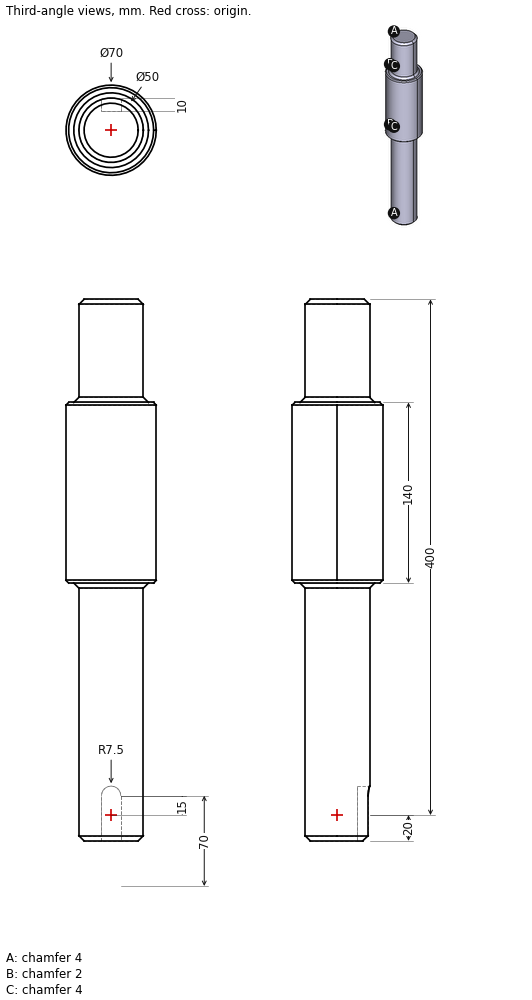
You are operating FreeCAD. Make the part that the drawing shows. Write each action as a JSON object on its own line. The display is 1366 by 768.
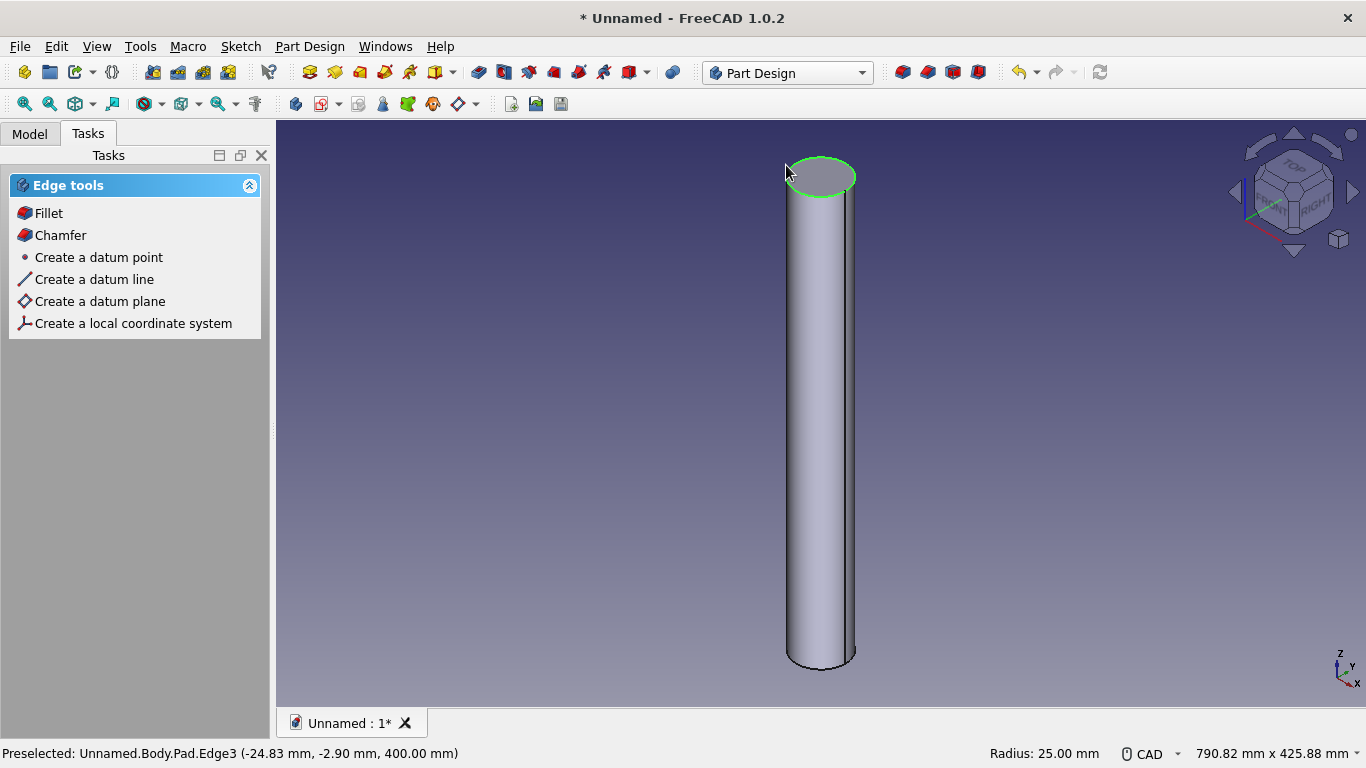
{"action": "left_click", "coordinate": [805, 667], "text": "ctrl"}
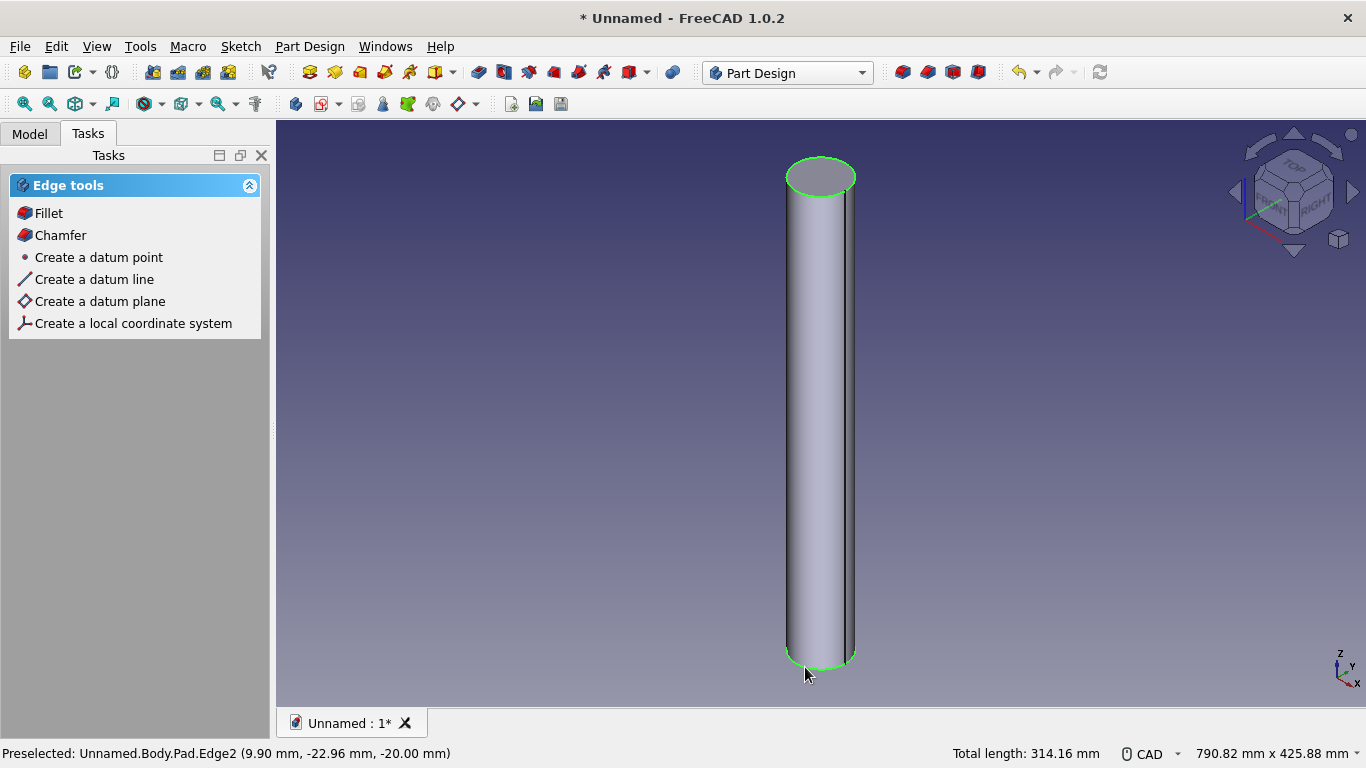
{"action": "left_click", "coordinate": [928, 72]}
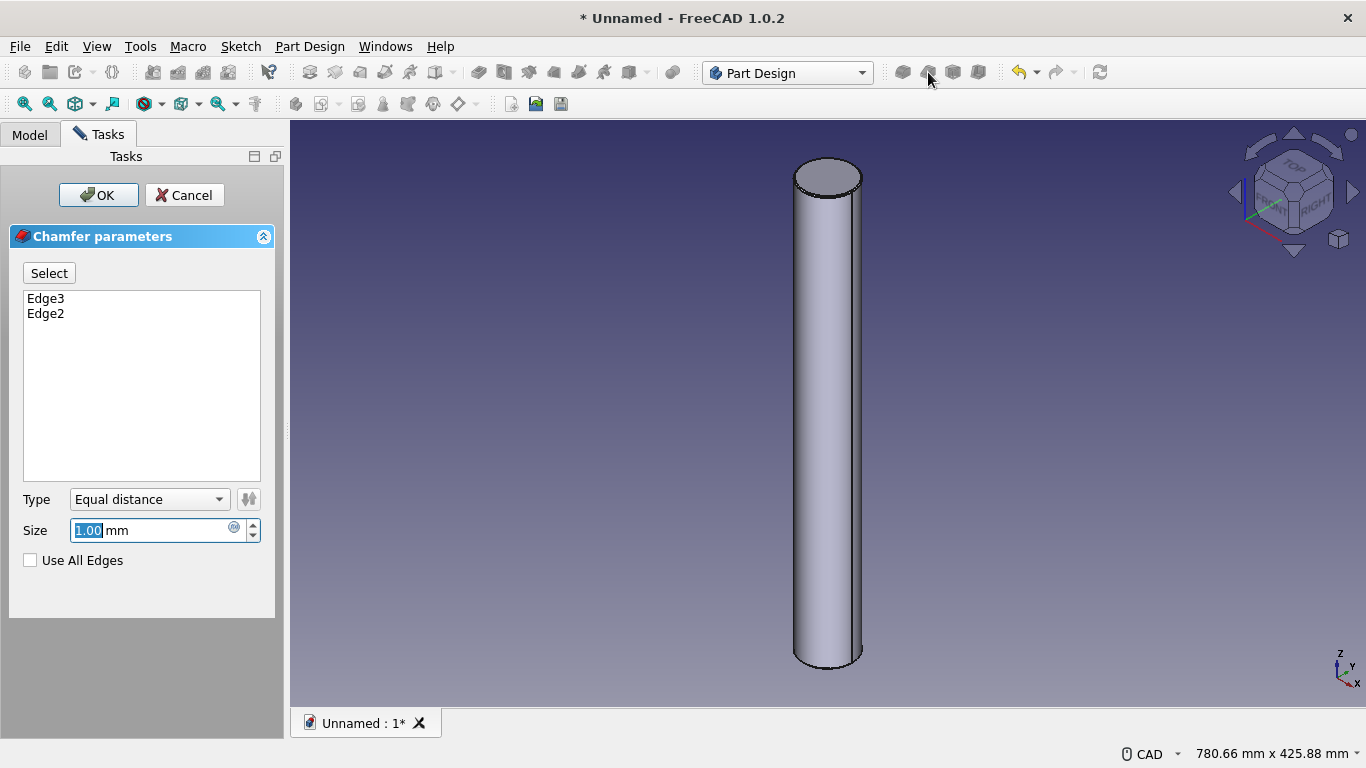
{"action": "type", "text": "4"}
{"action": "key", "text": "Tab"}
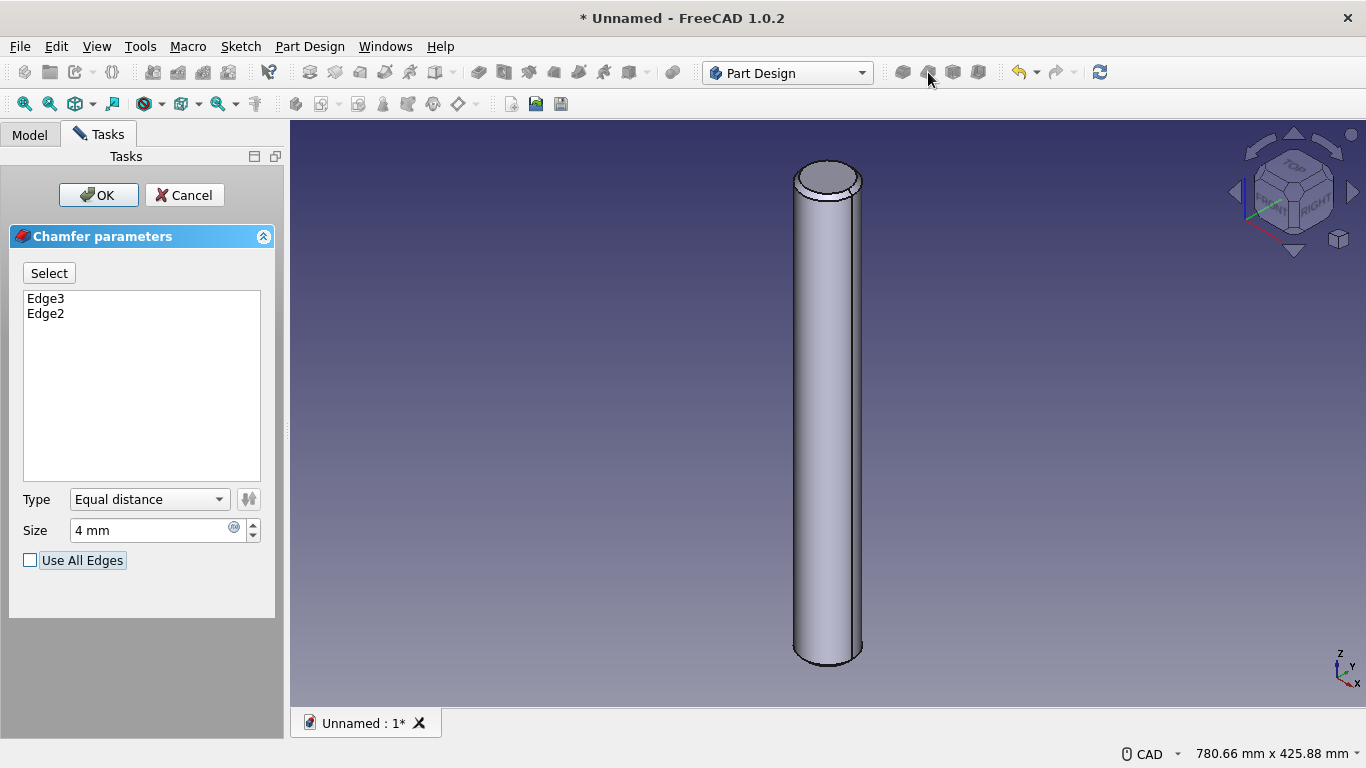
{"action": "left_click", "coordinate": [99, 195]}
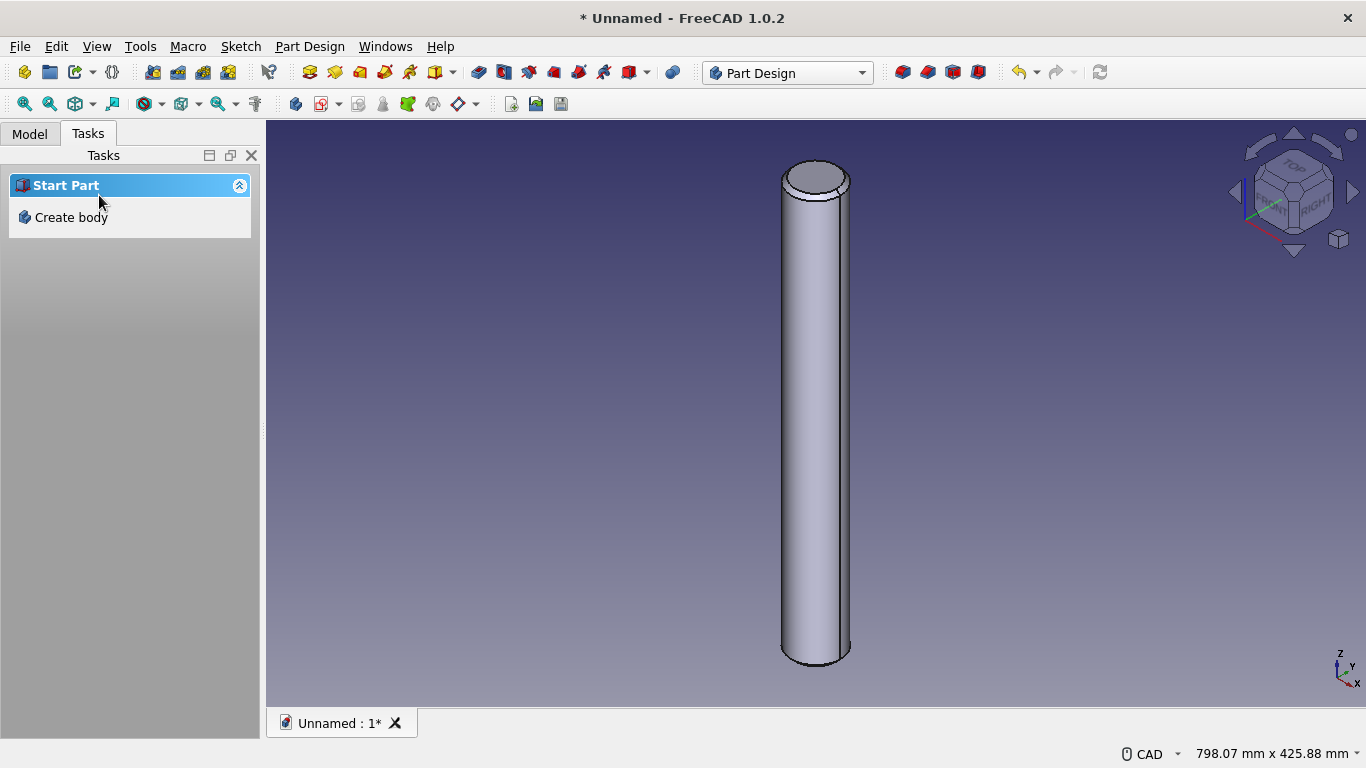
{"action": "left_click", "coordinate": [30, 134]}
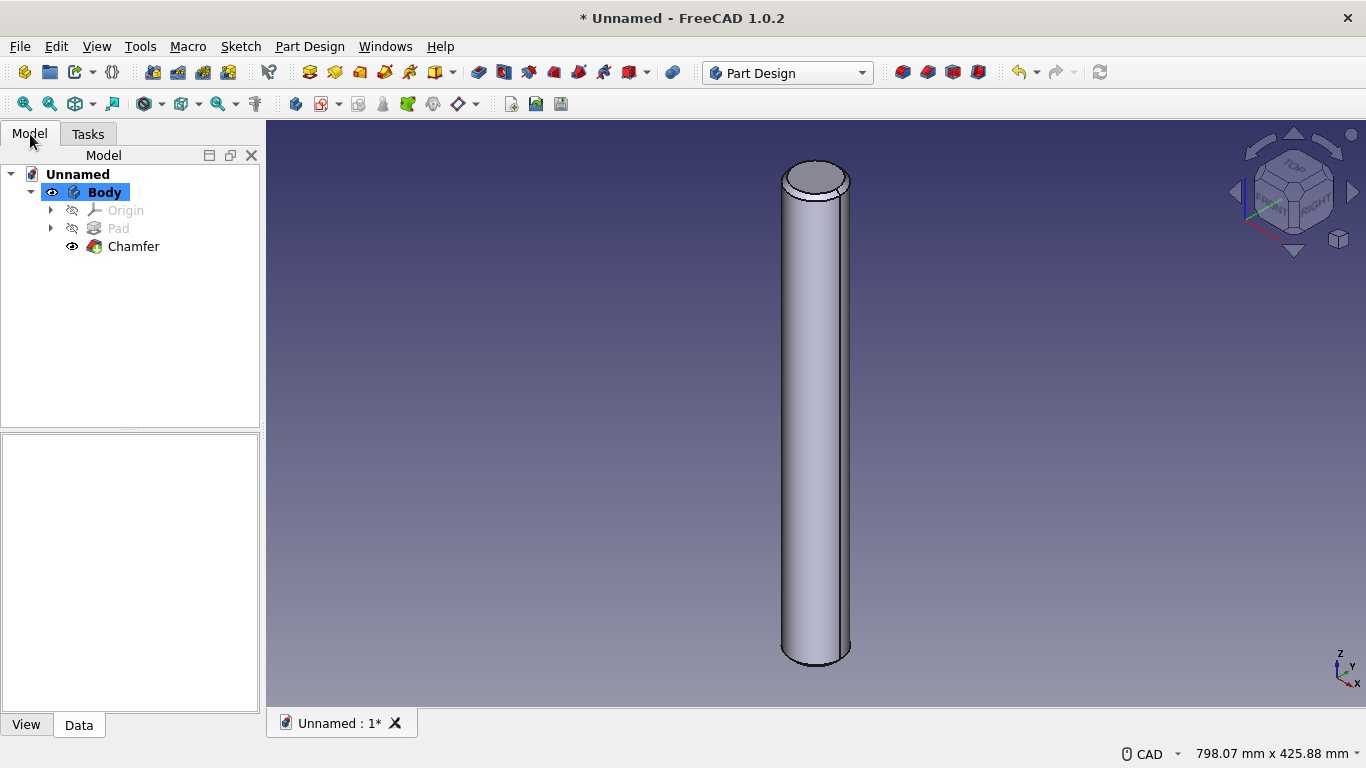
{"action": "left_click", "coordinate": [51, 210]}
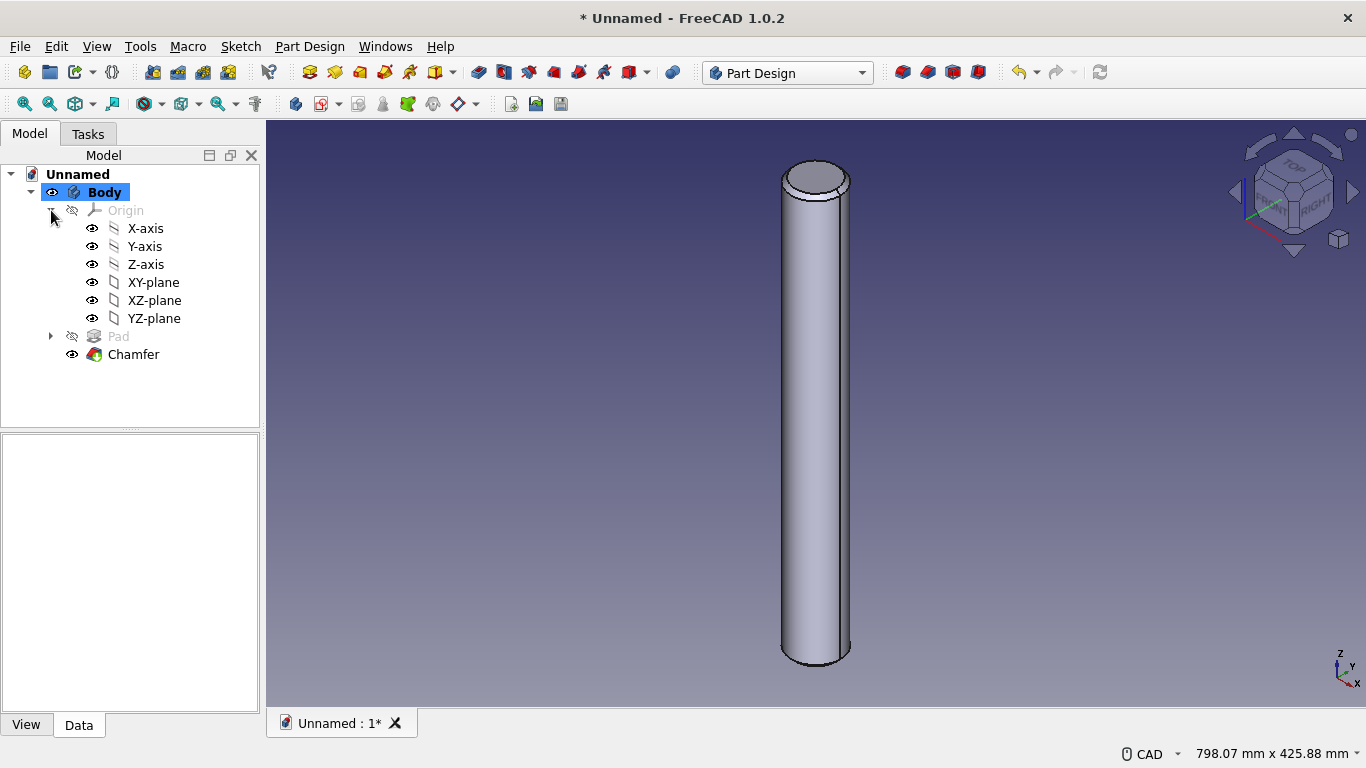
{"action": "left_click", "coordinate": [137, 300]}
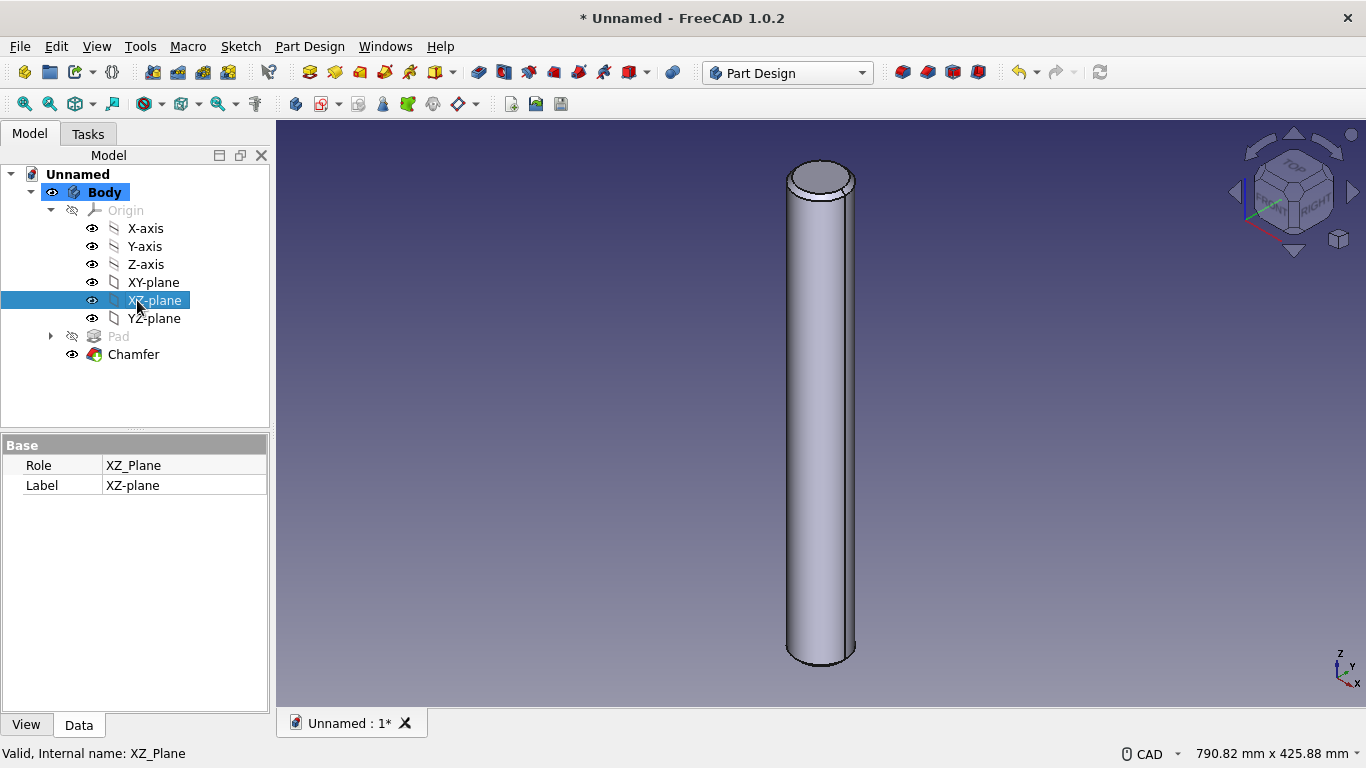
{"action": "left_click", "coordinate": [458, 104]}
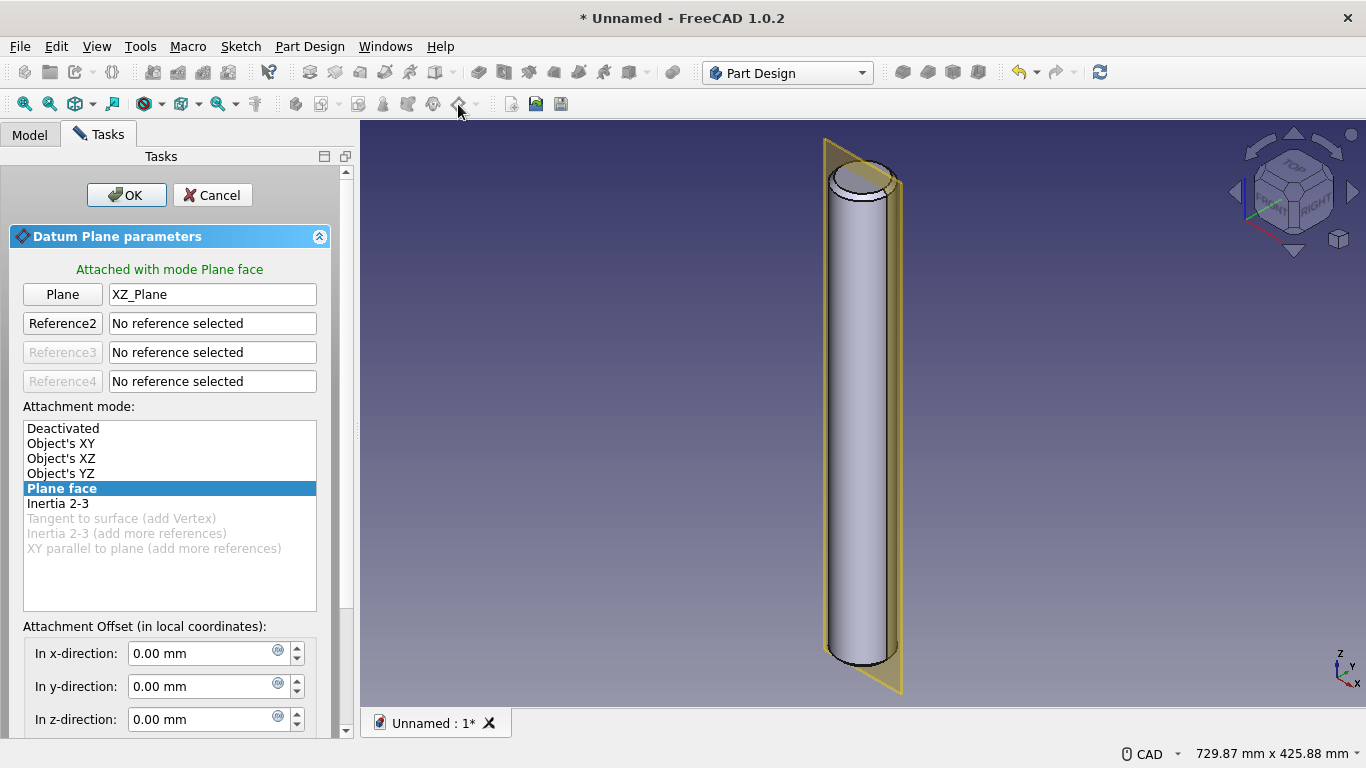
{"action": "triple_click", "coordinate": [210, 720]}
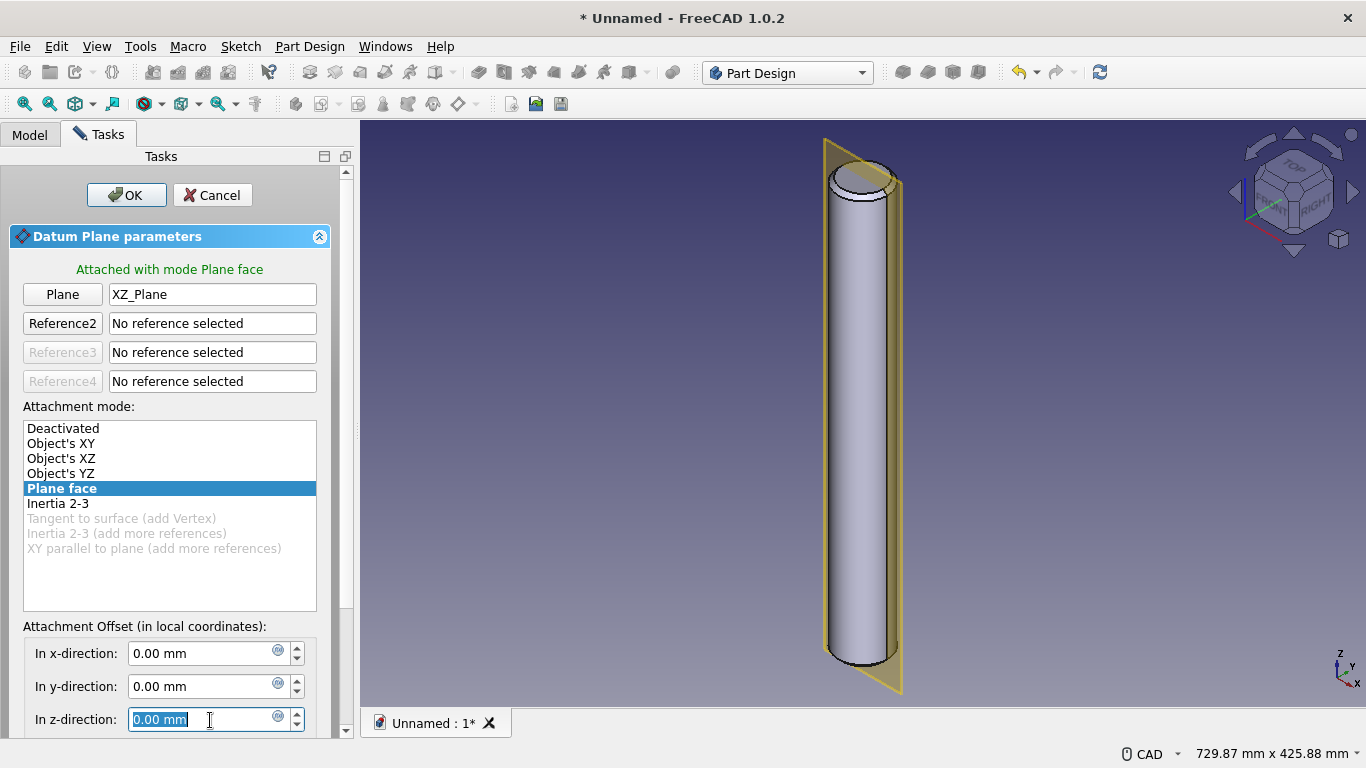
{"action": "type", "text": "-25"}
{"action": "key", "text": "Tab"}